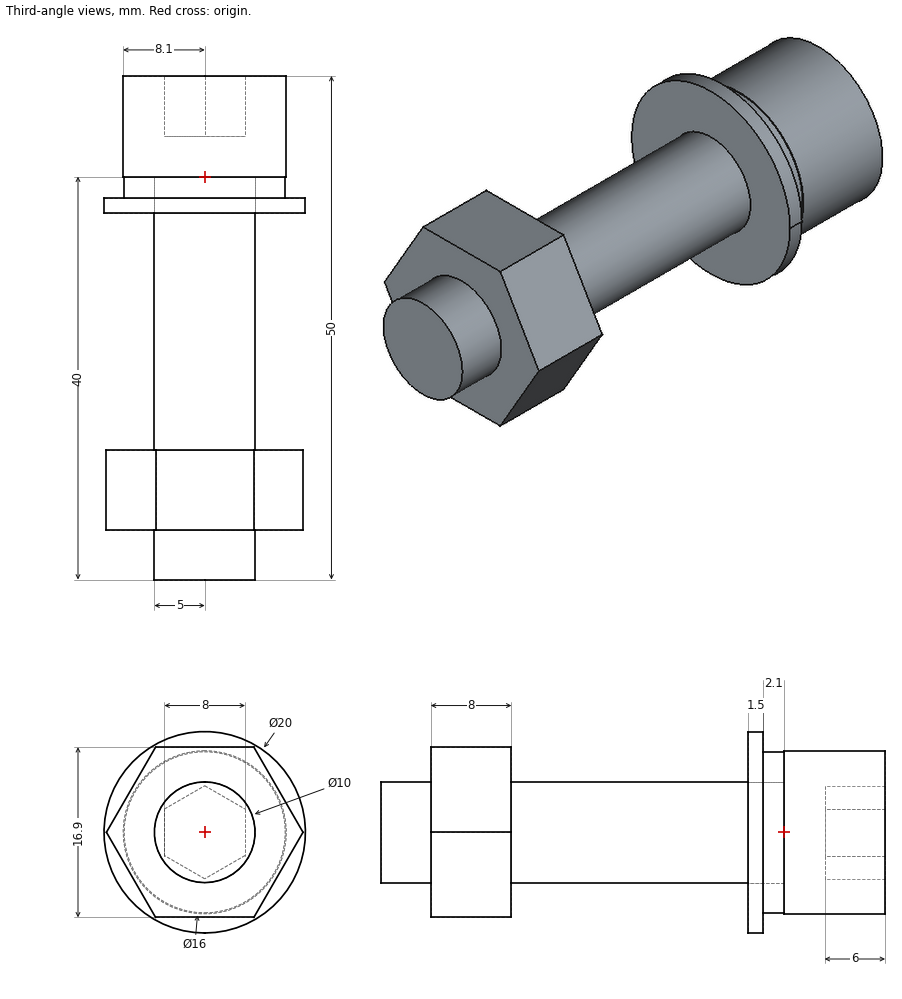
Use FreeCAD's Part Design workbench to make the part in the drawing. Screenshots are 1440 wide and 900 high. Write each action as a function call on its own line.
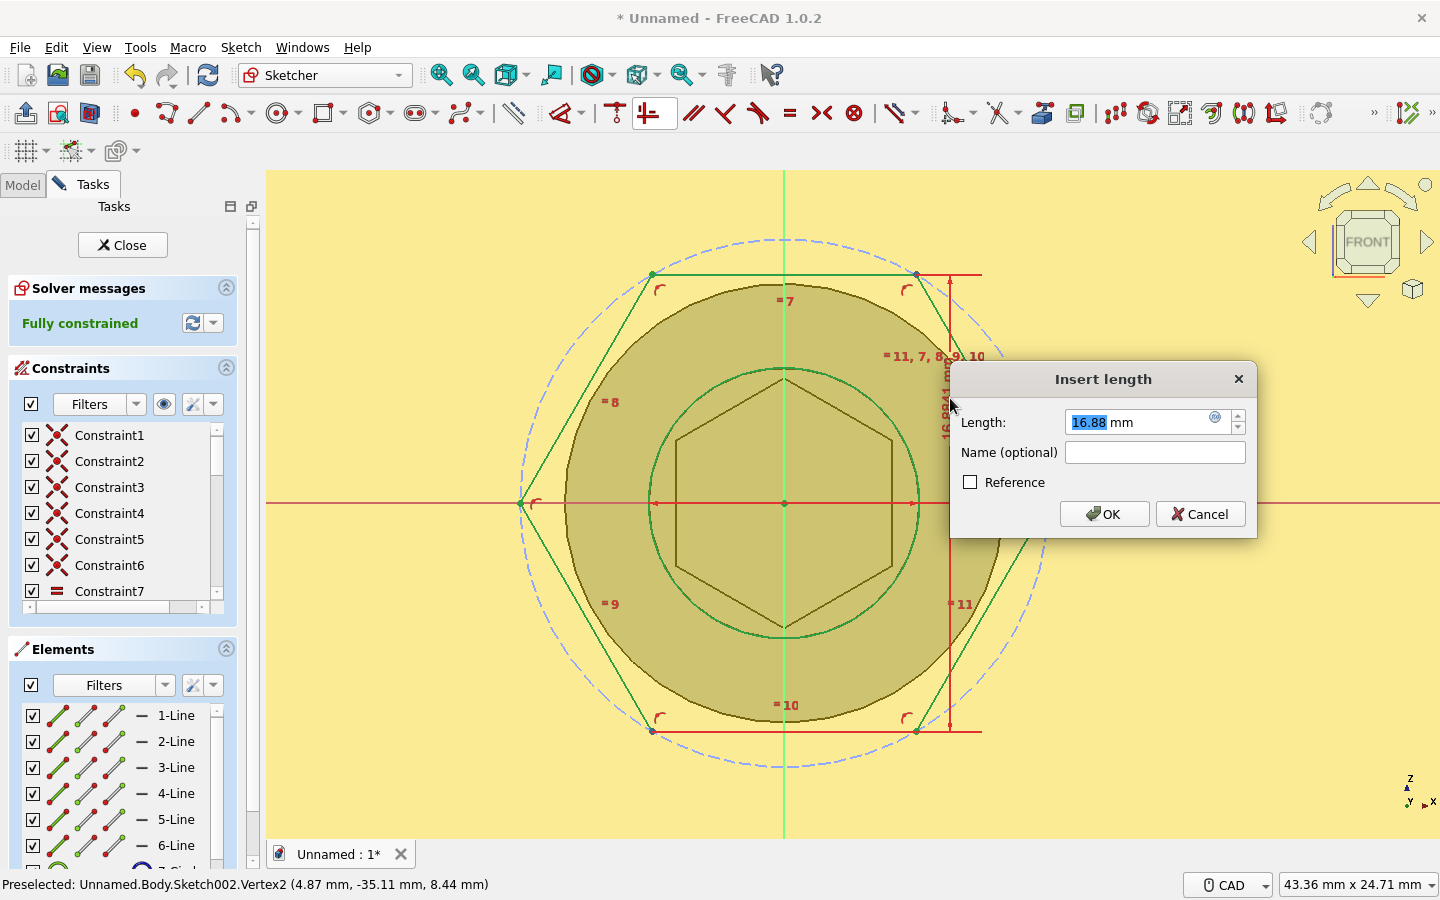
text(16.9)
key(Return)
key(Escape)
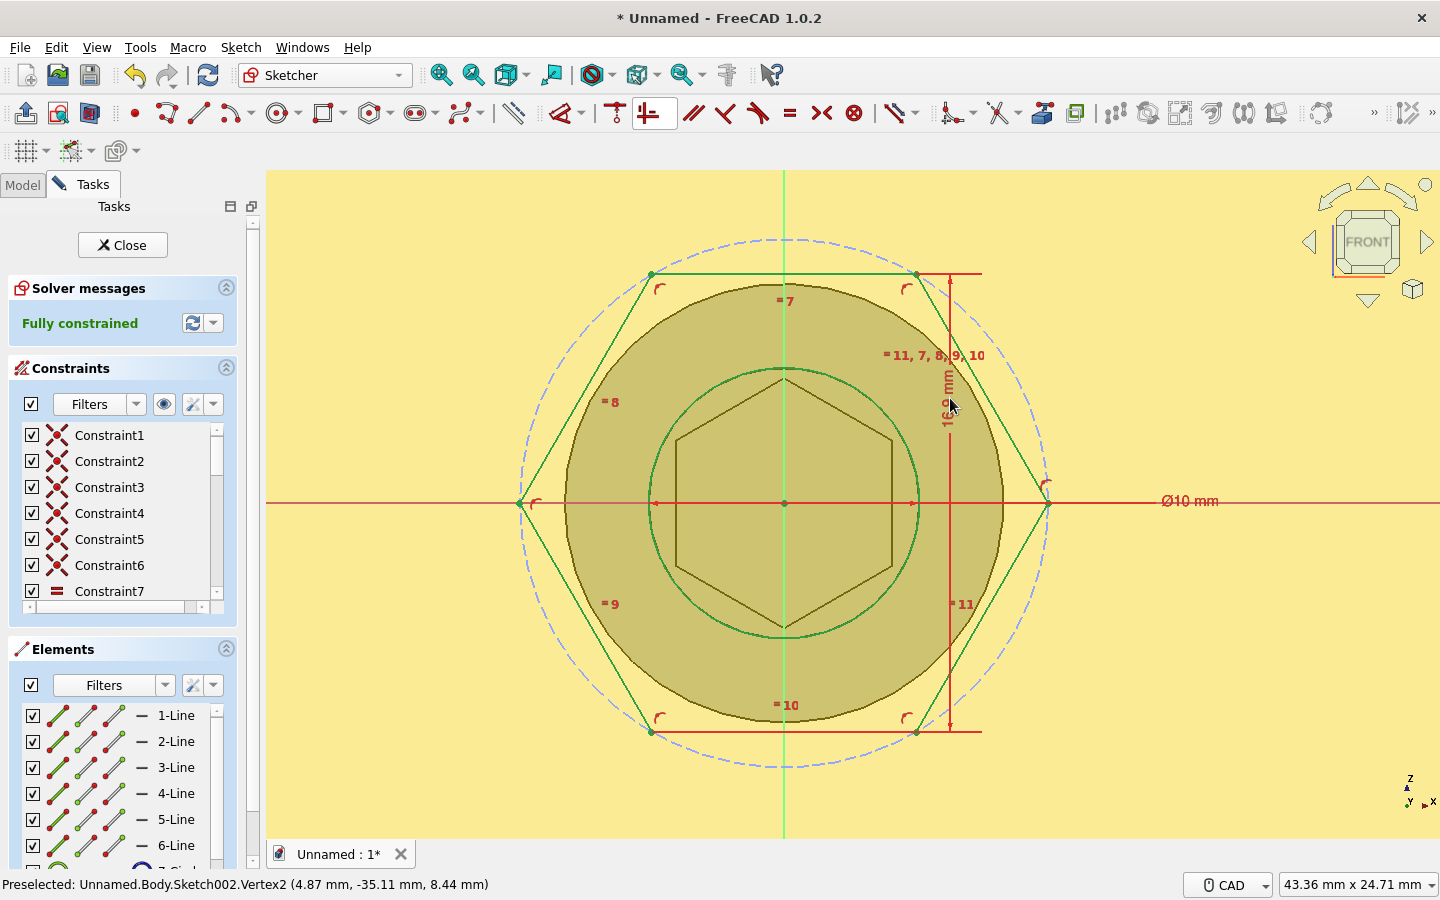
click(123, 245)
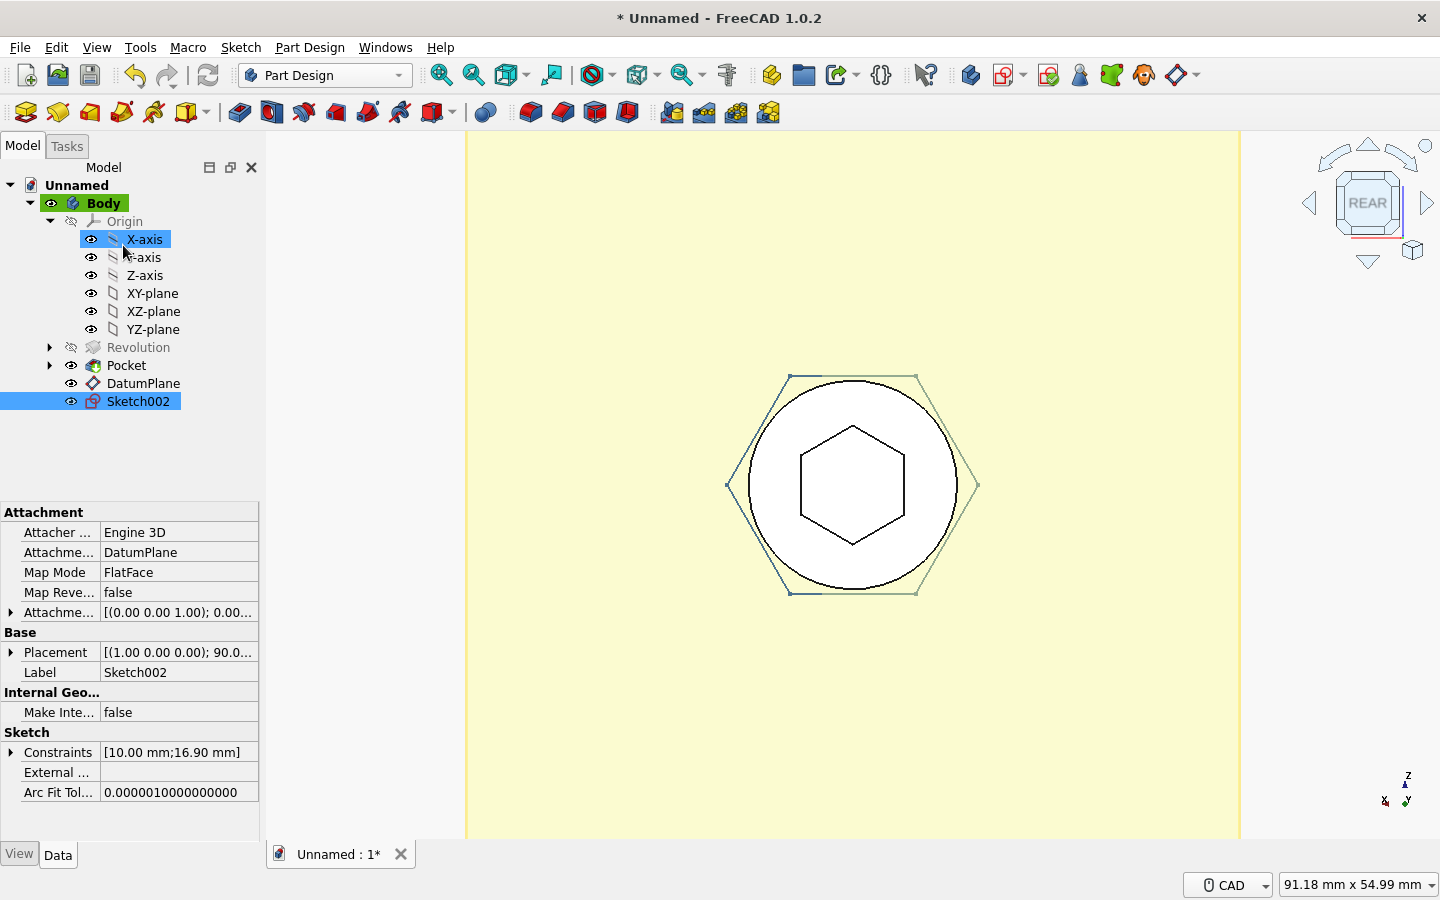
click(26, 112)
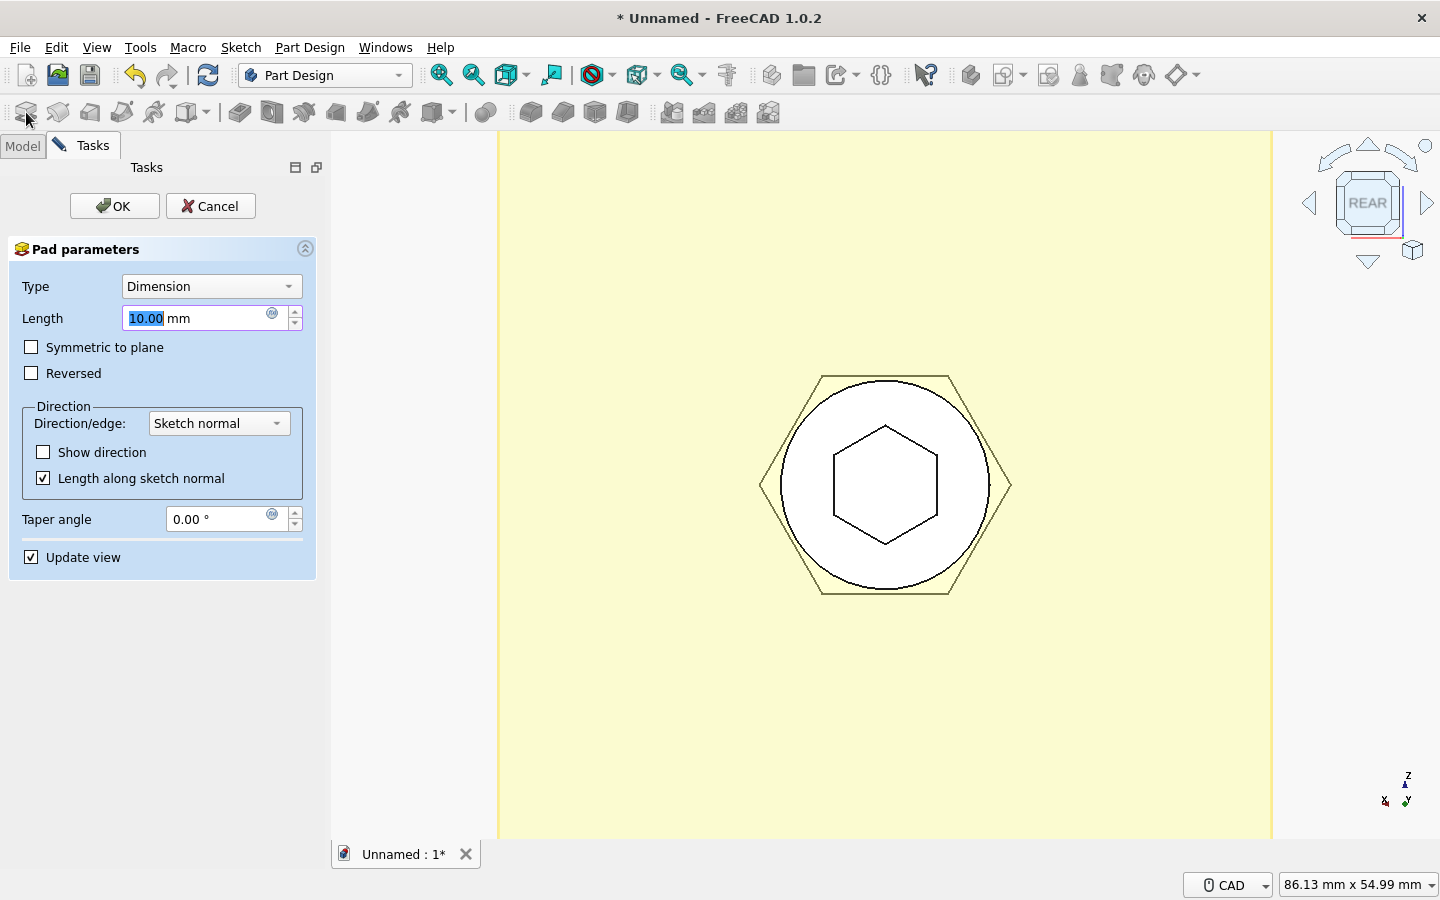
text(8)
key(Tab)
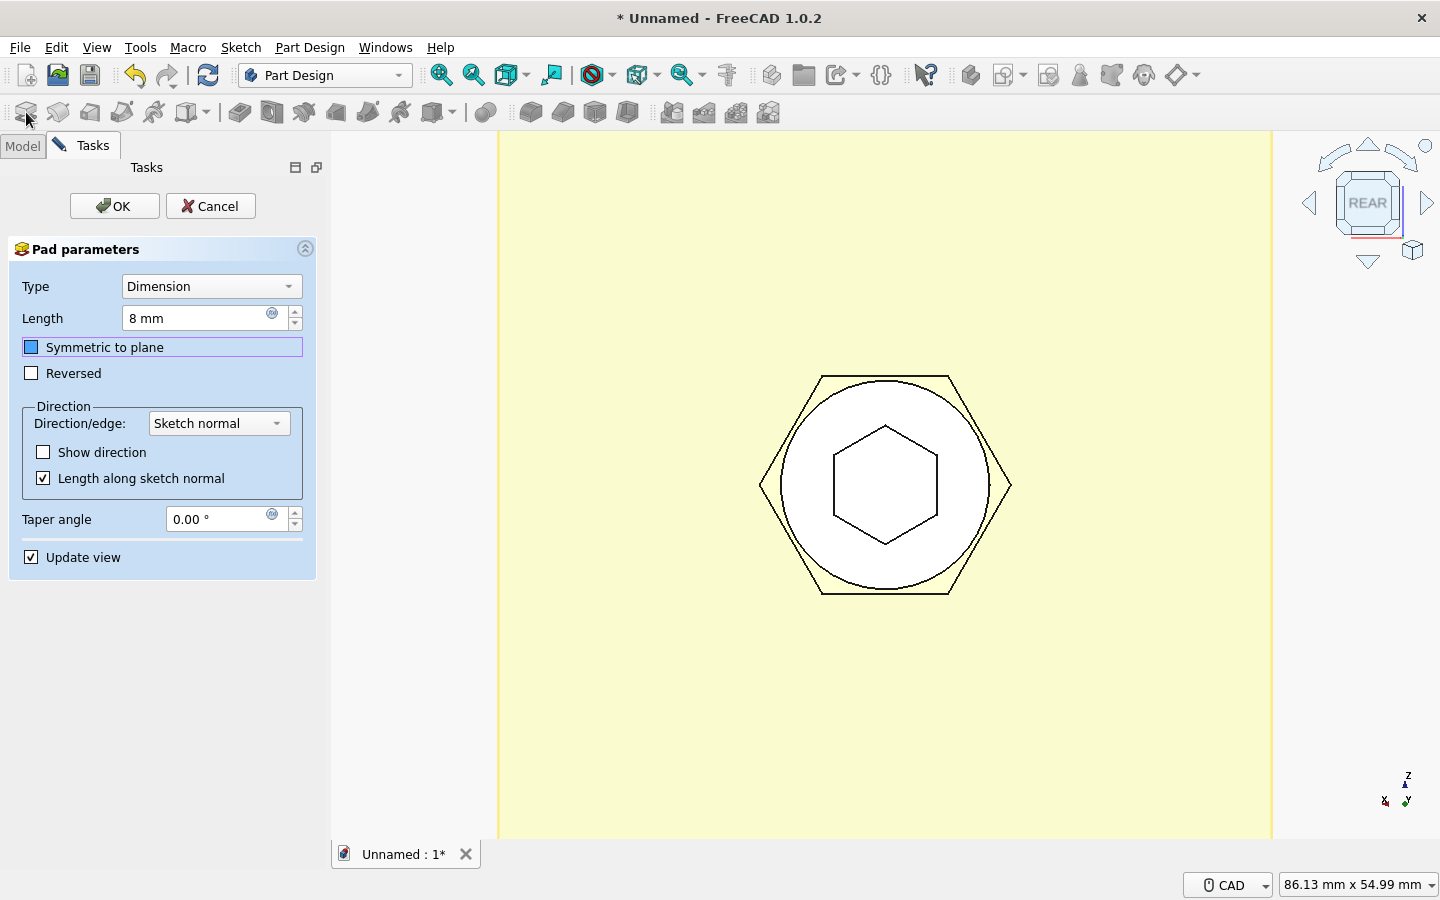
click(30, 373)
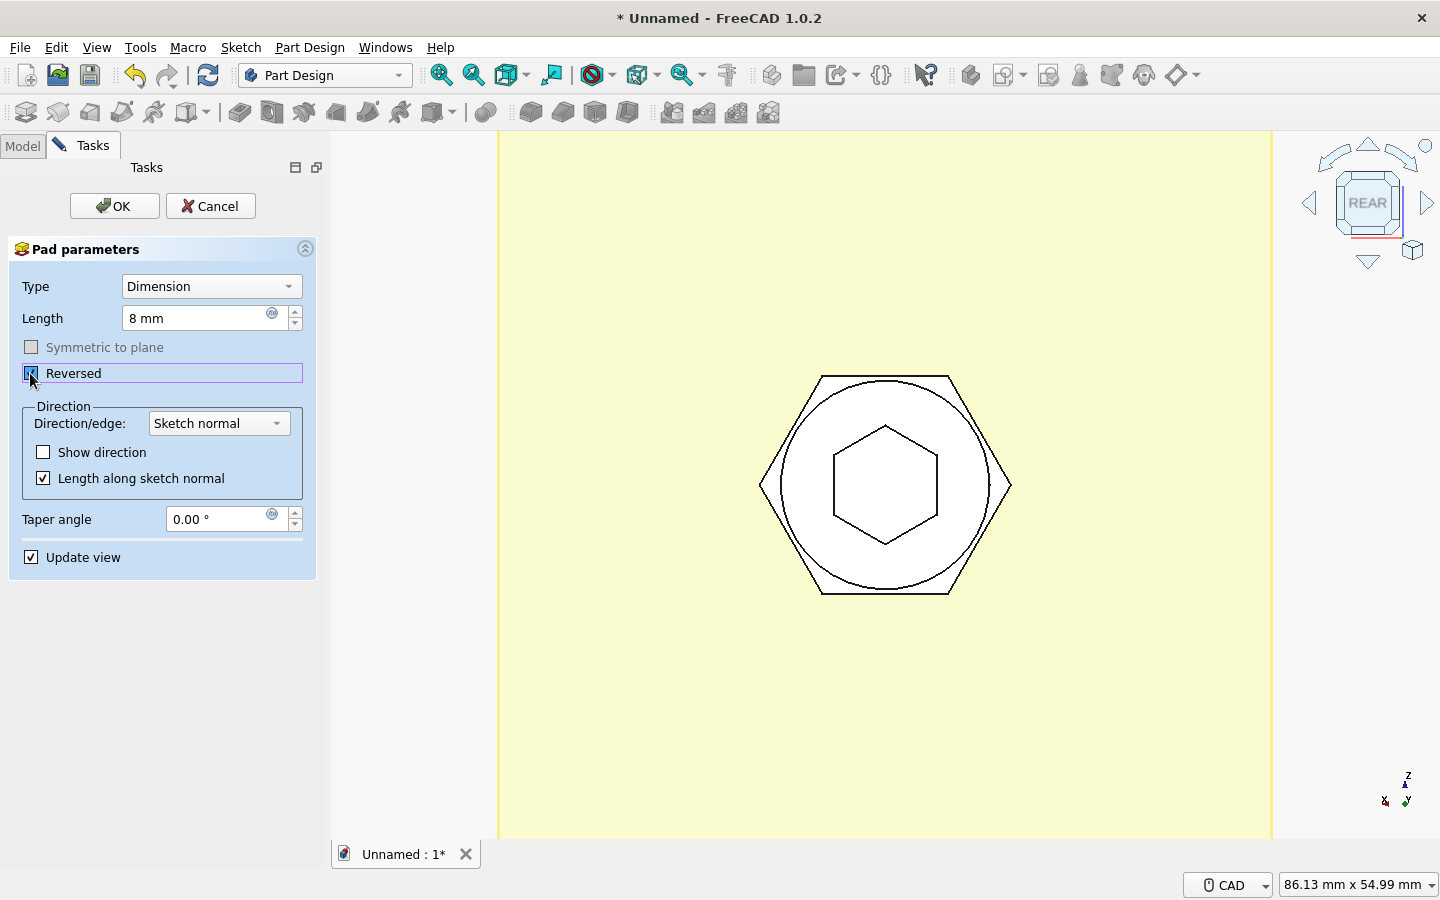
click(115, 206)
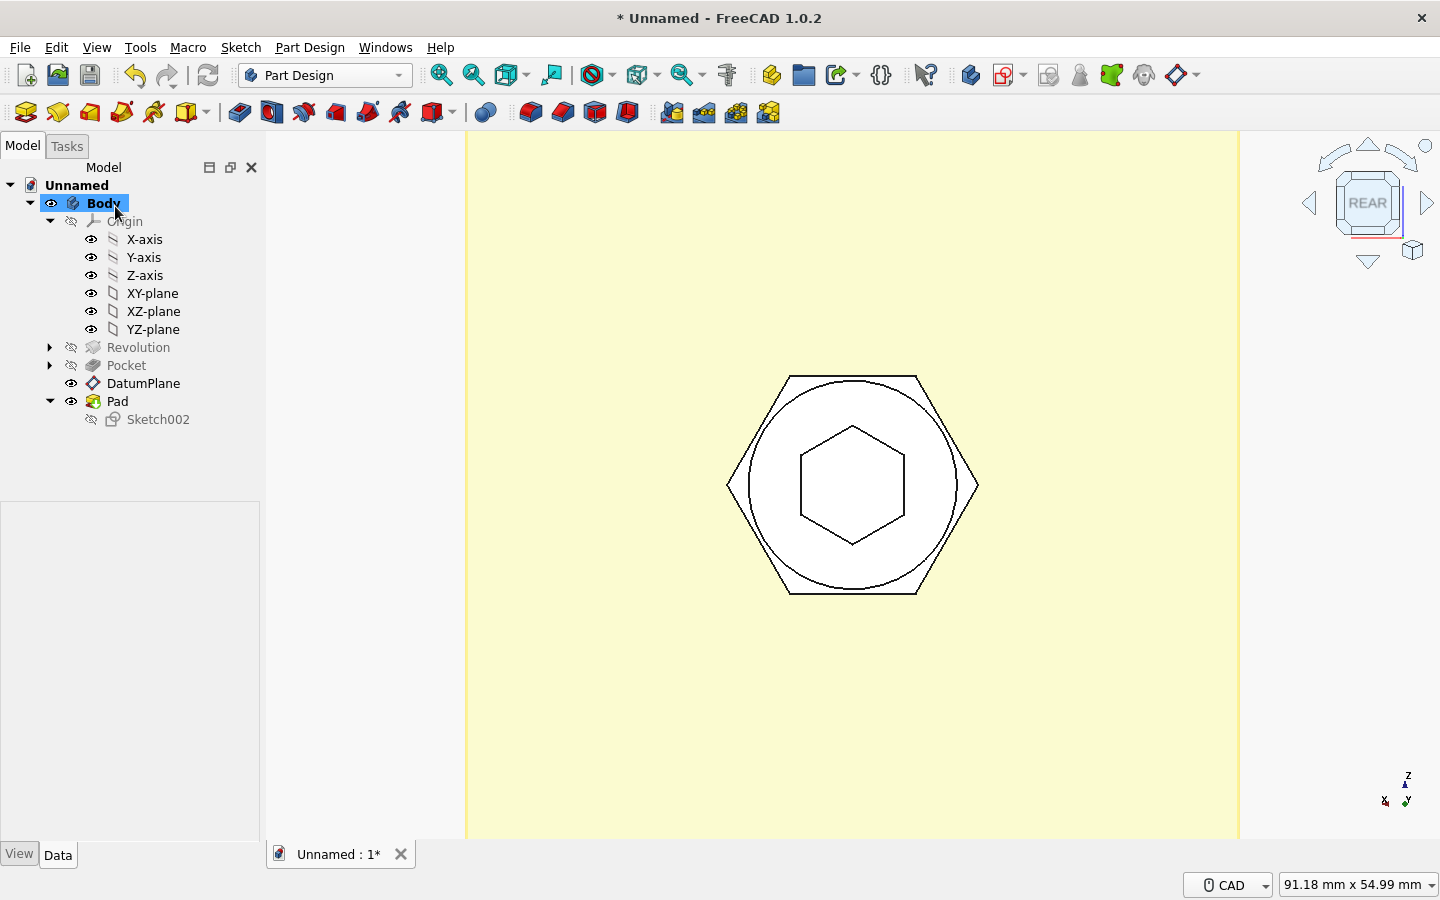
click(116, 383)
key(space)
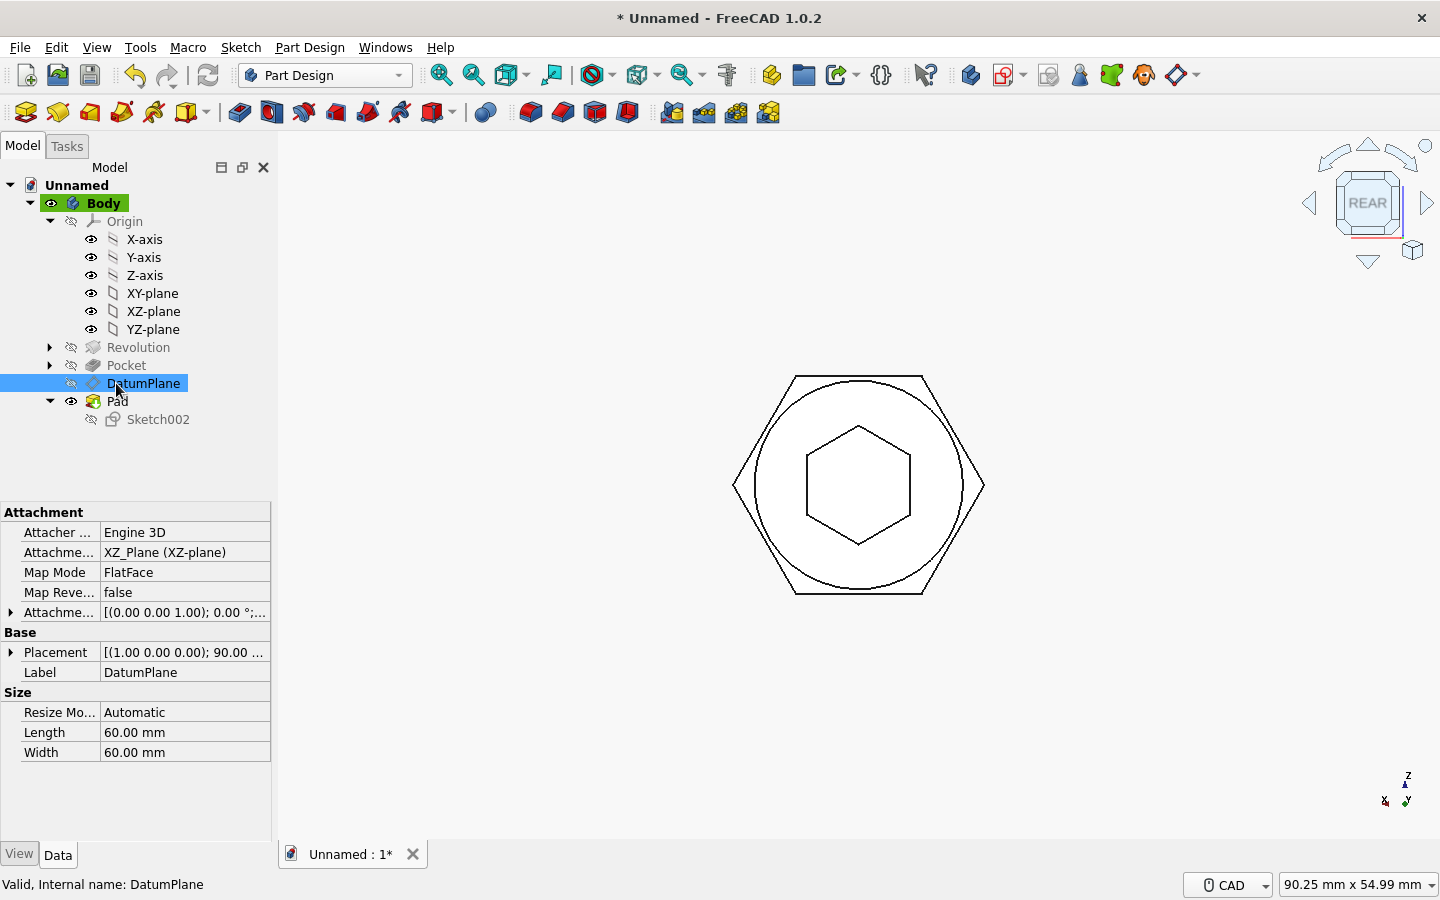
click(442, 76)